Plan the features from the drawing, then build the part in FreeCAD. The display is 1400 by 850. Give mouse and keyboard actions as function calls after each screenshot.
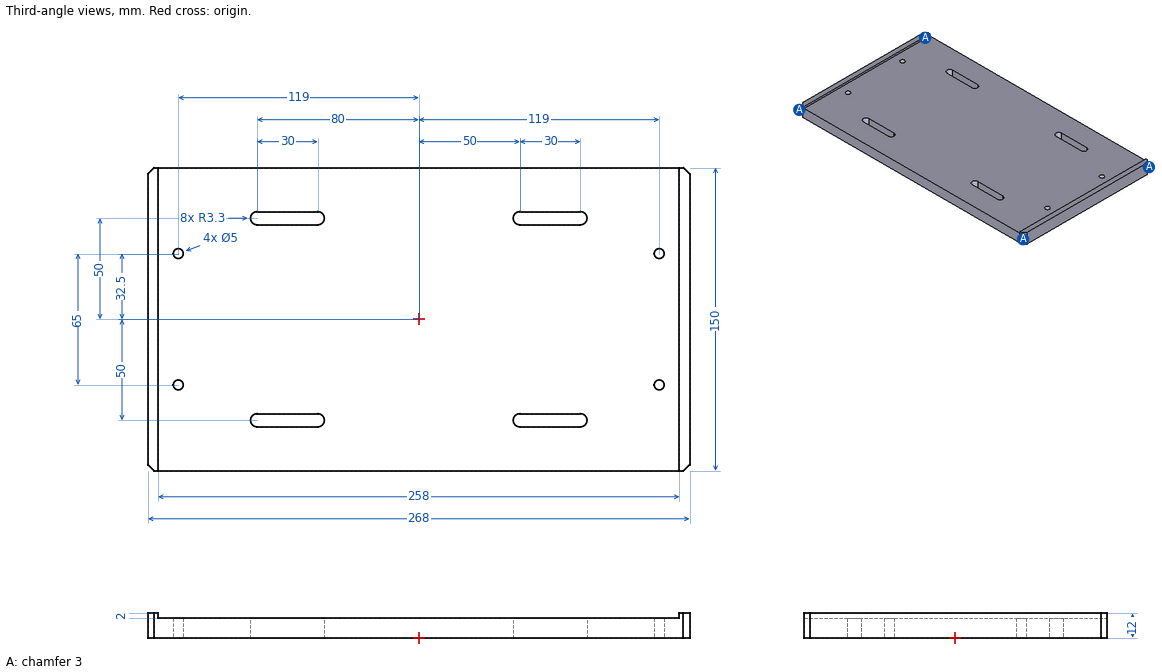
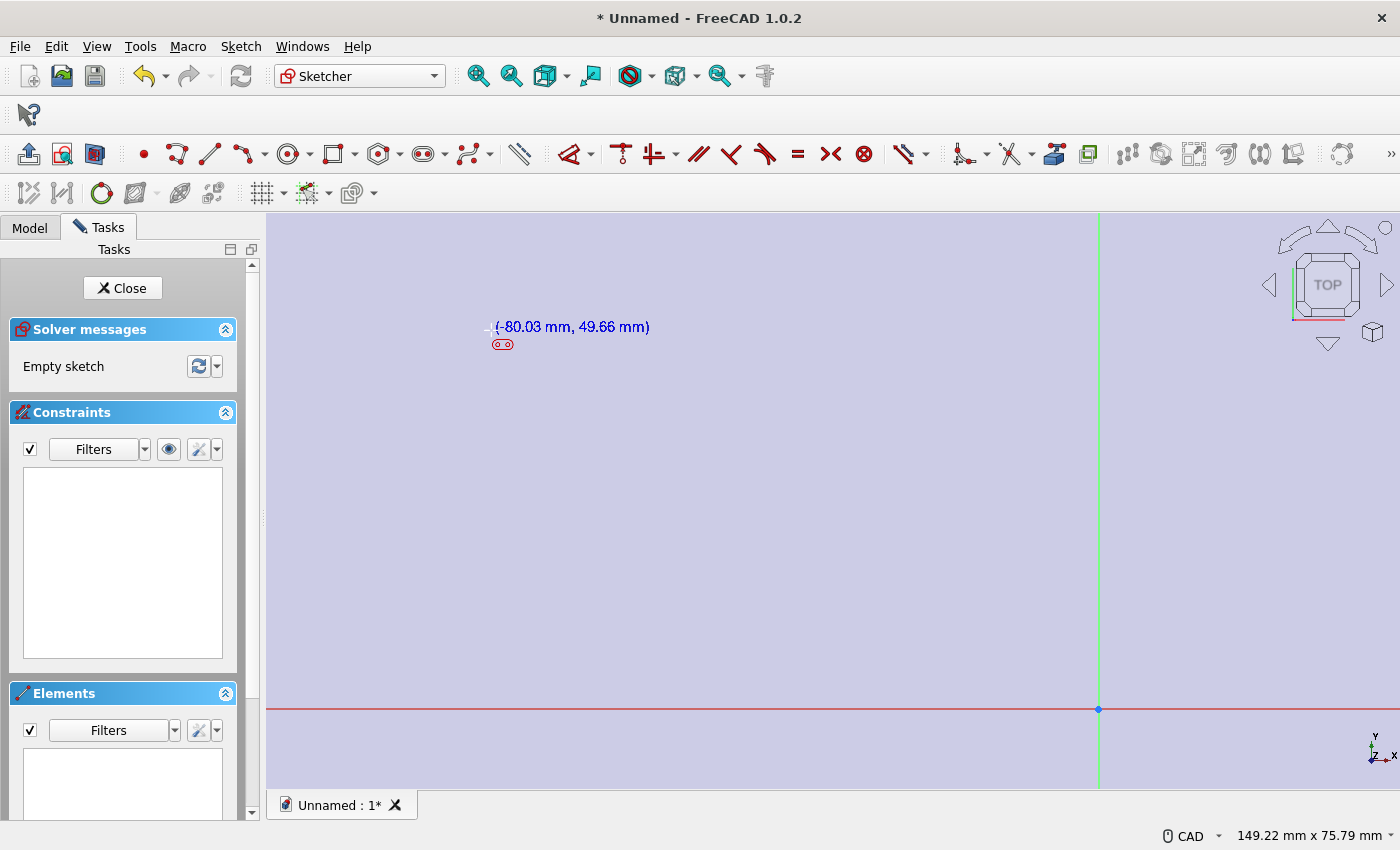
click(491, 329)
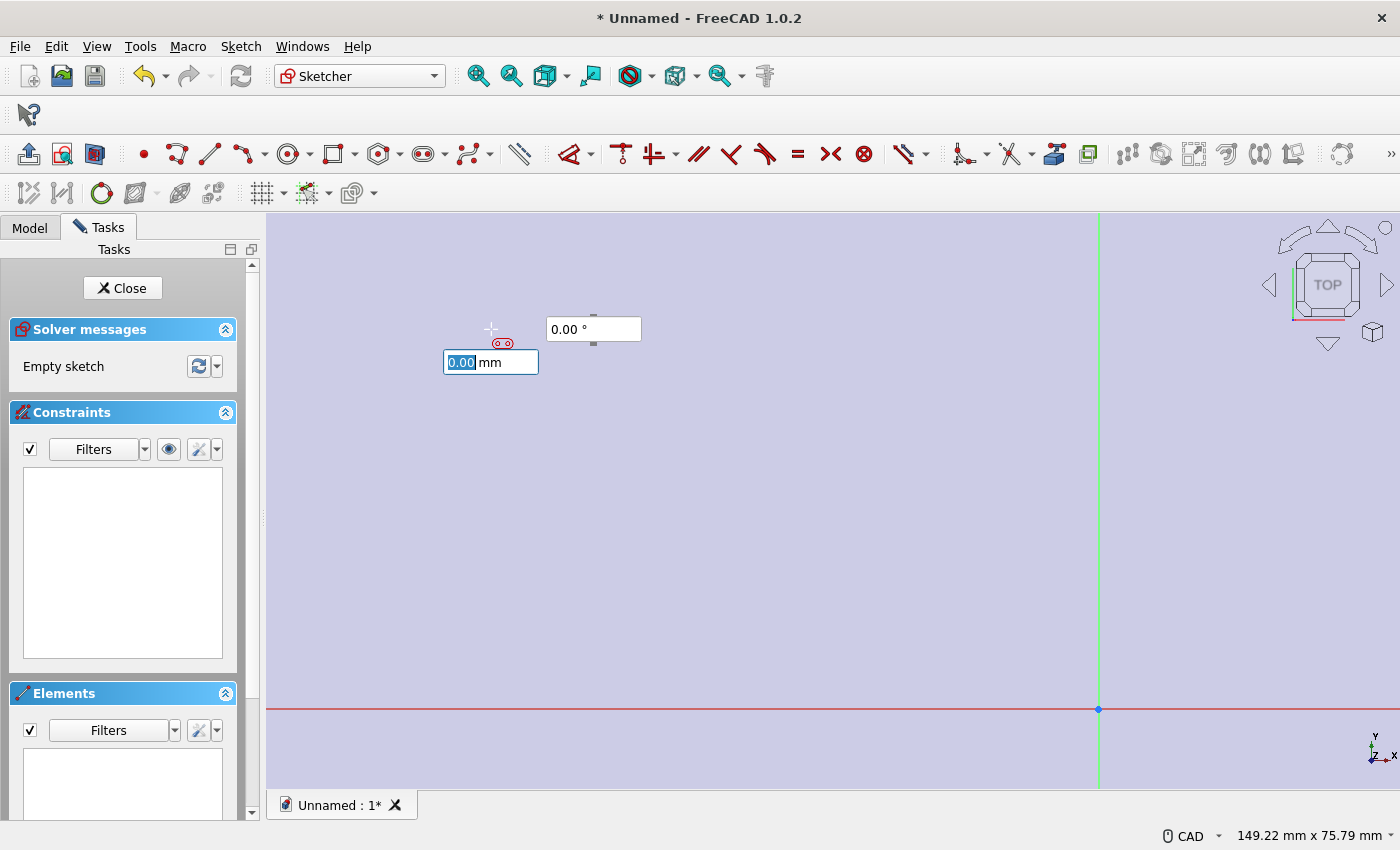
click(719, 329)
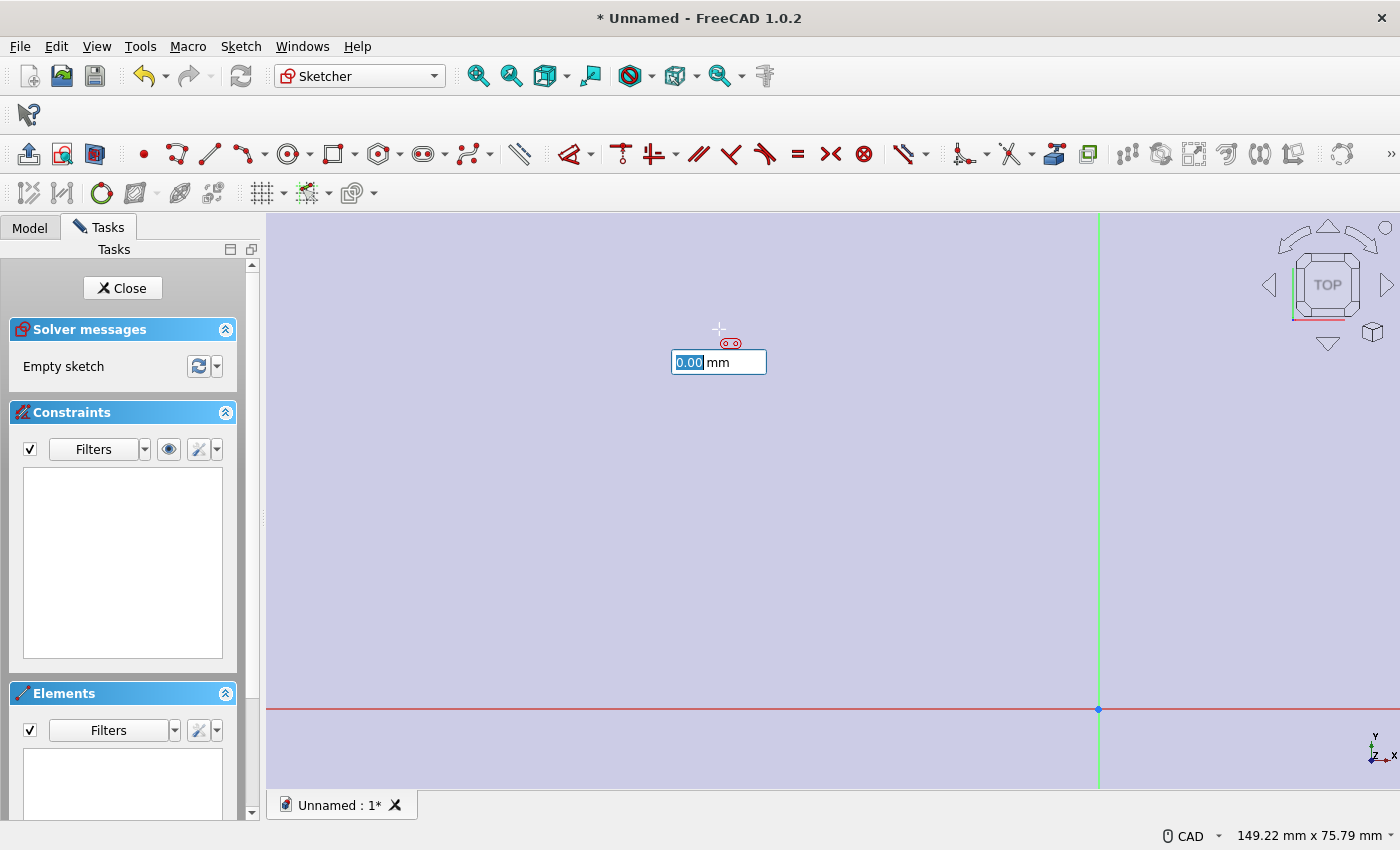
click(605, 304)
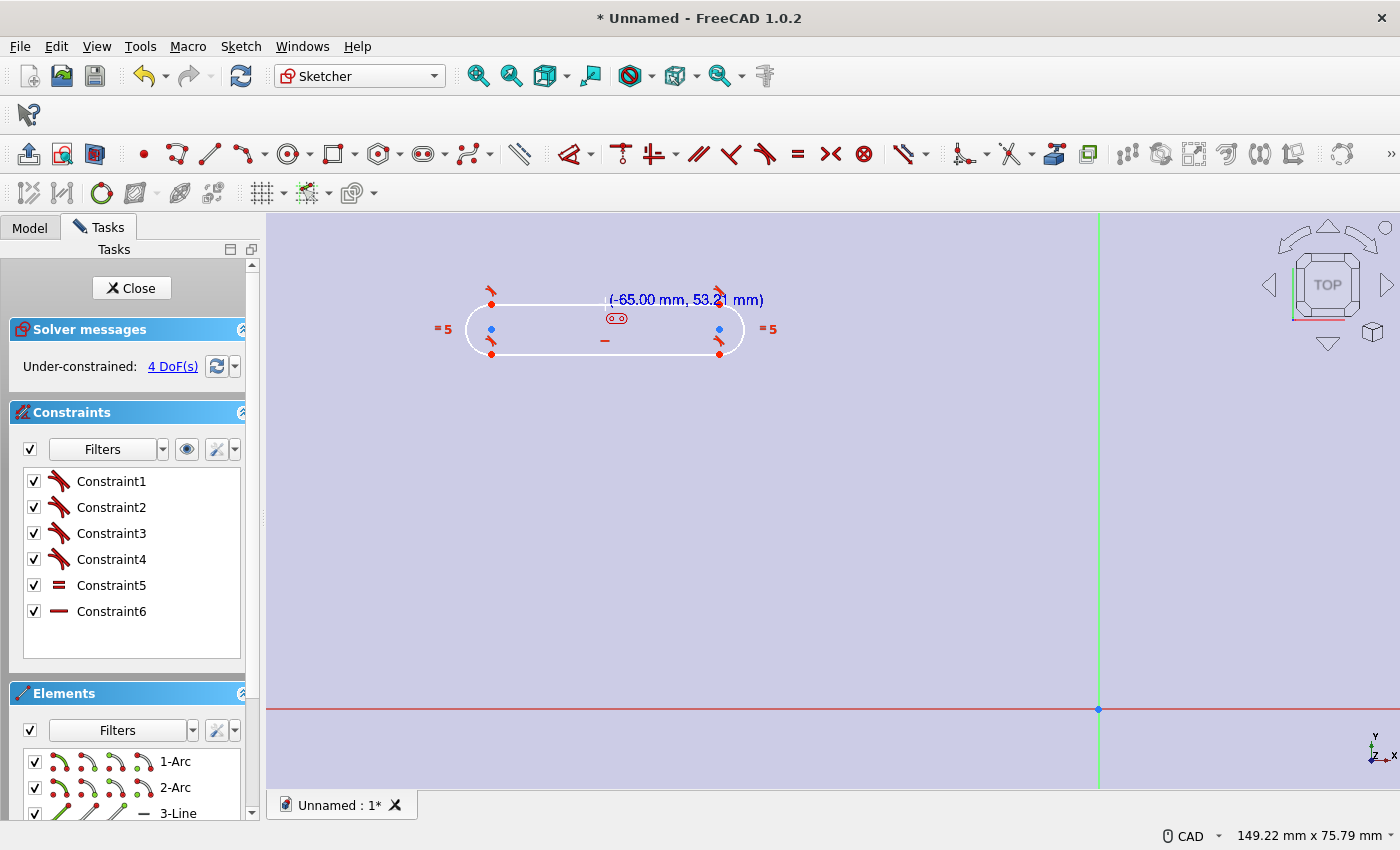
scroll(492, 331, down, 4)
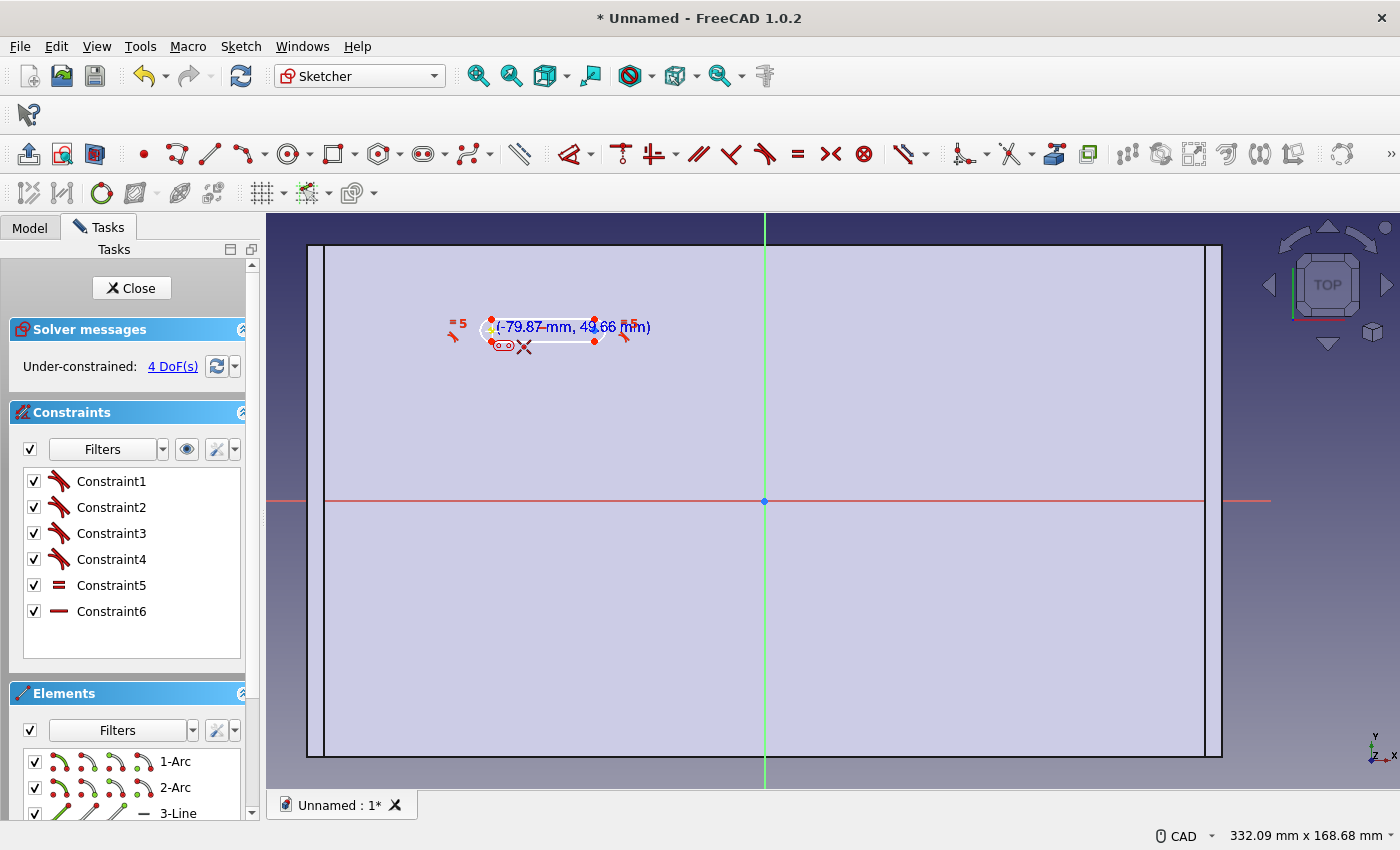
scroll(936, 330, up, 4)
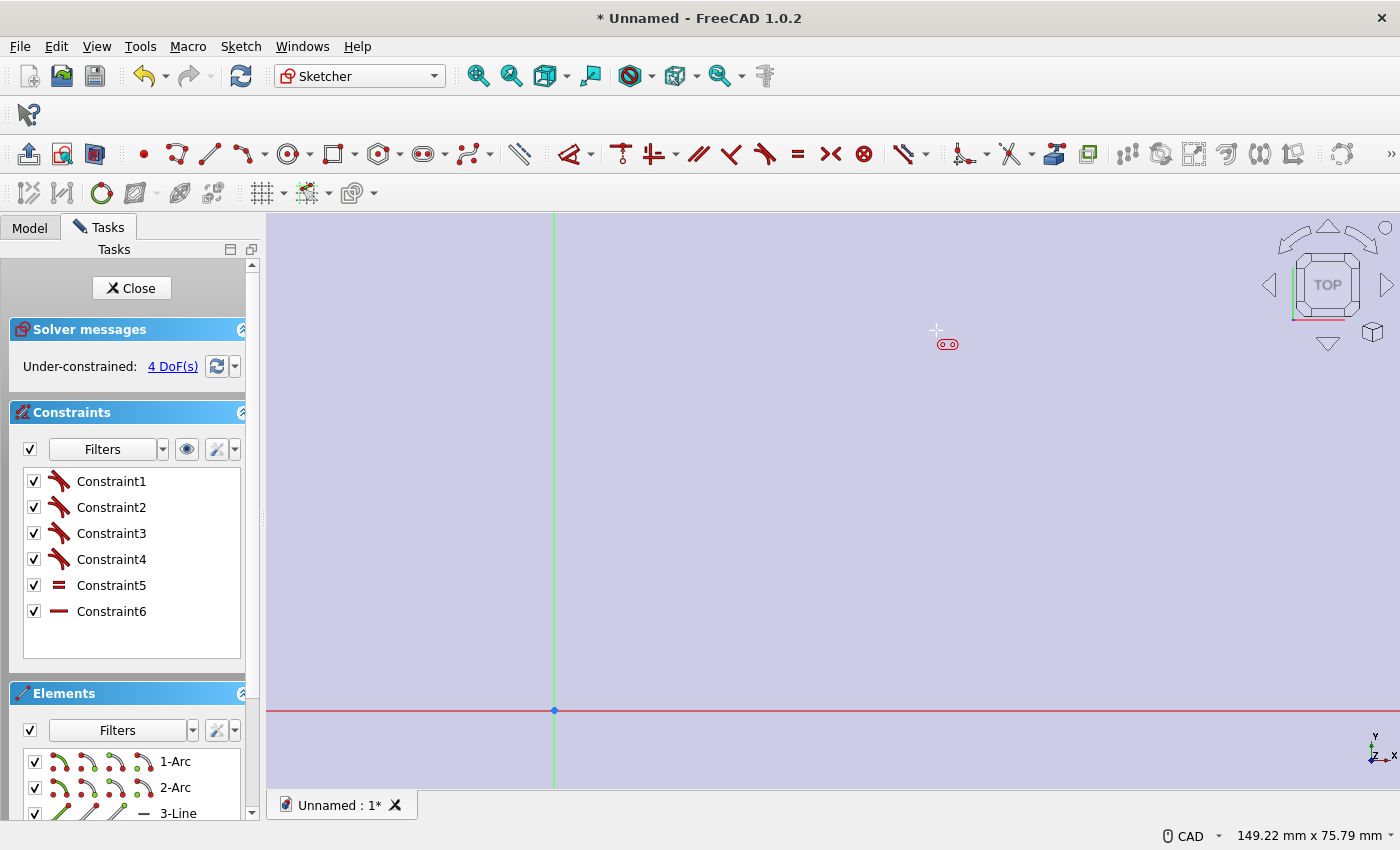
click(934, 331)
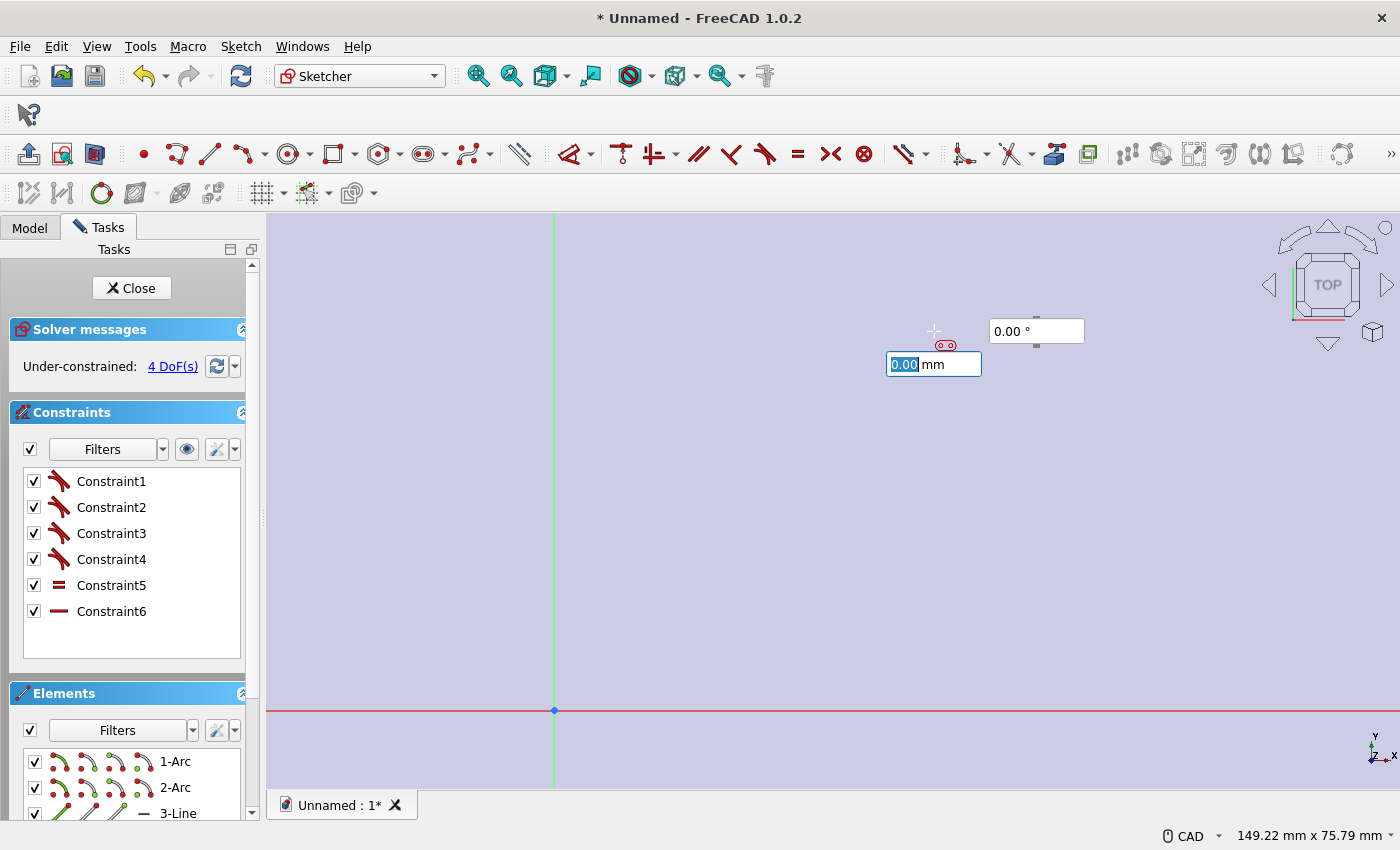
click(1162, 331)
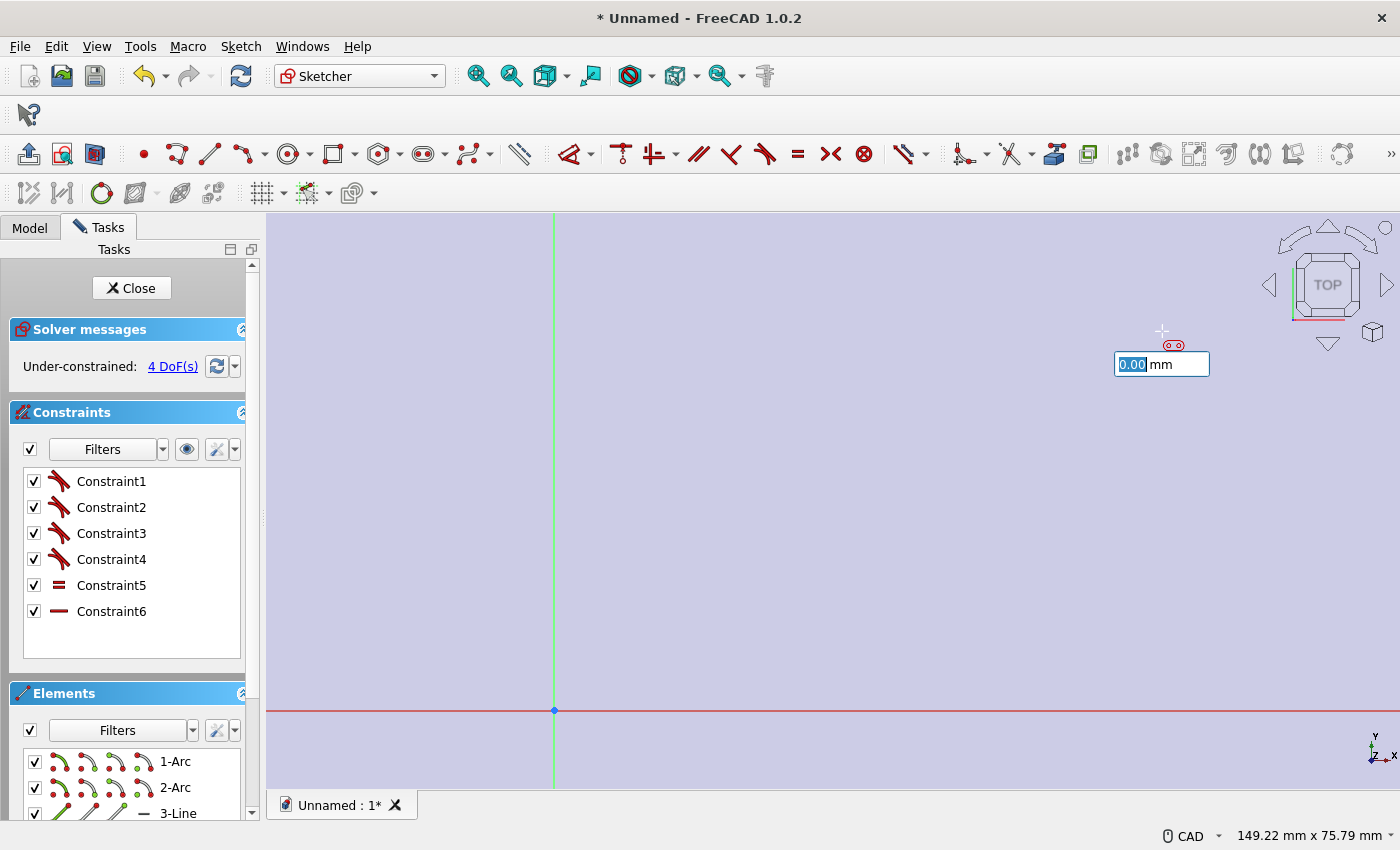
click(1048, 306)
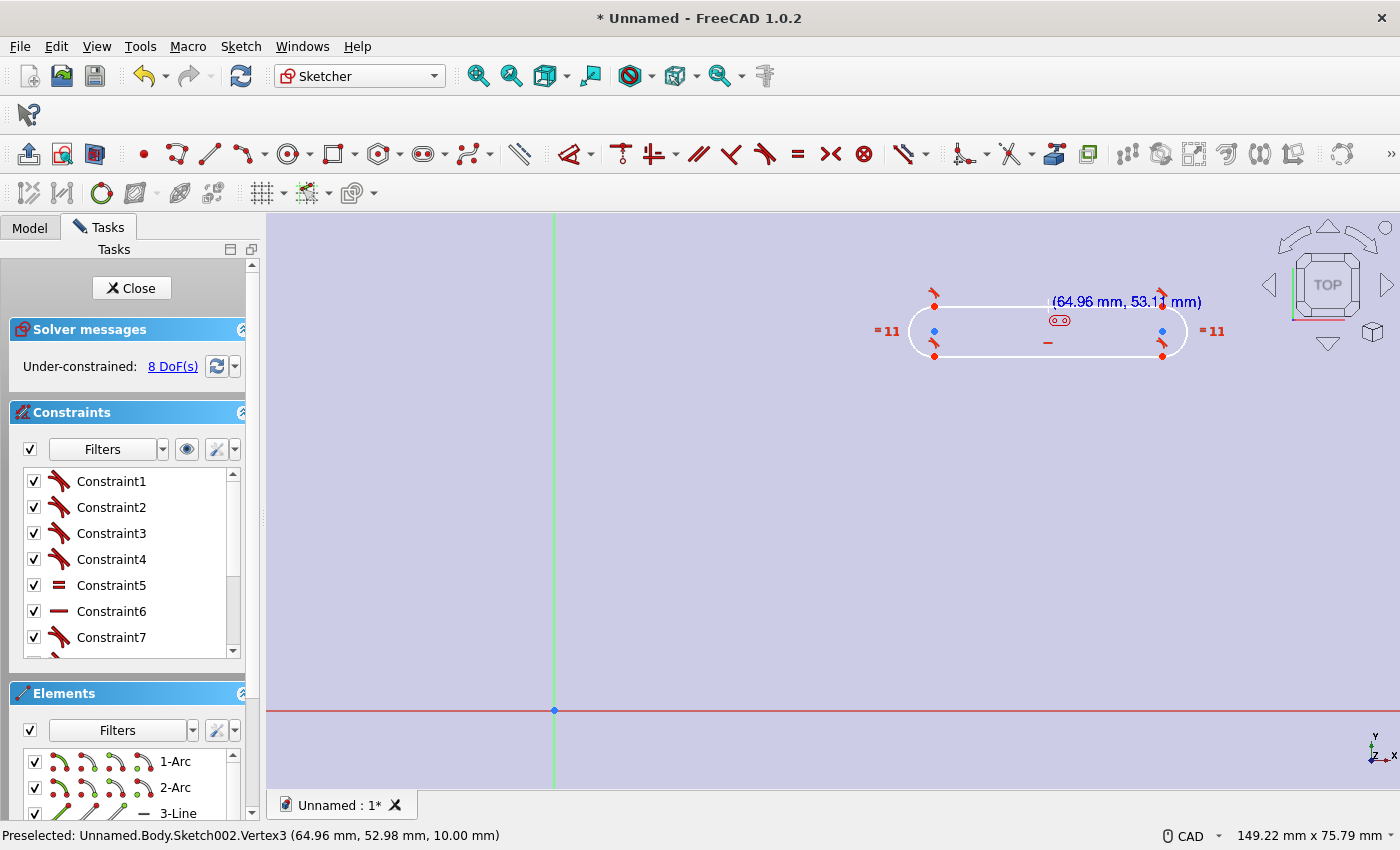
scroll(936, 330, down, 4)